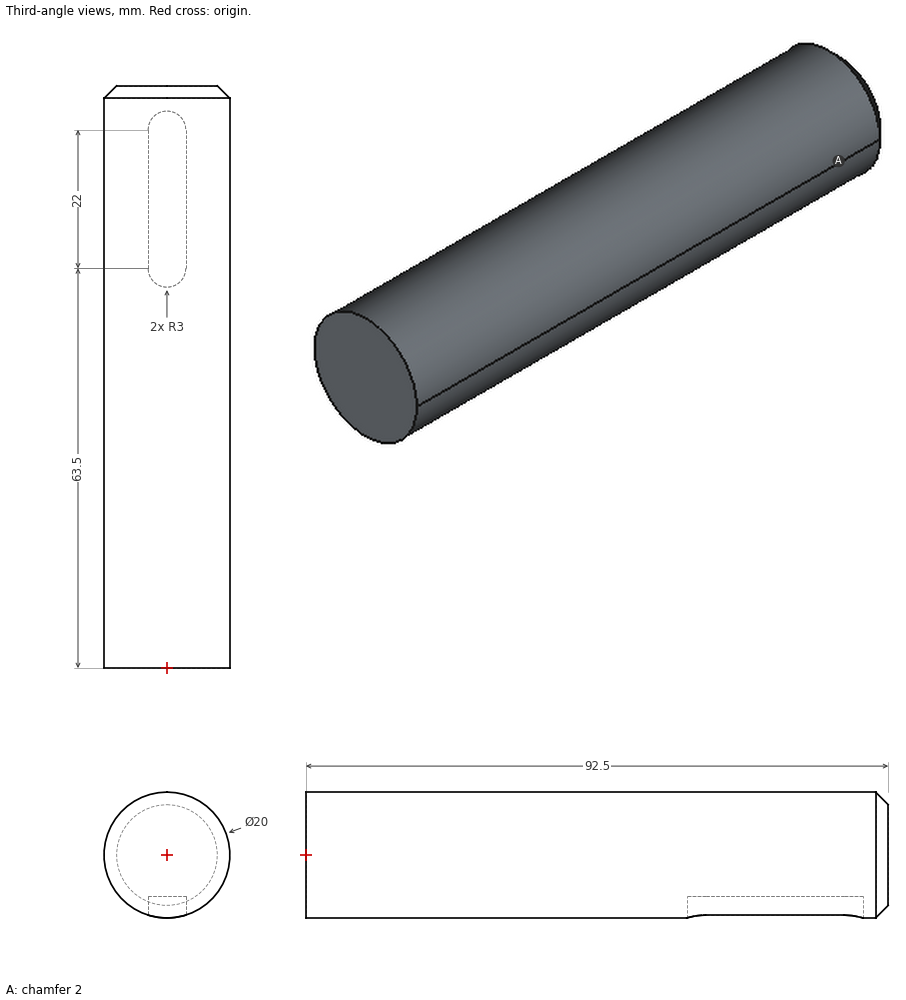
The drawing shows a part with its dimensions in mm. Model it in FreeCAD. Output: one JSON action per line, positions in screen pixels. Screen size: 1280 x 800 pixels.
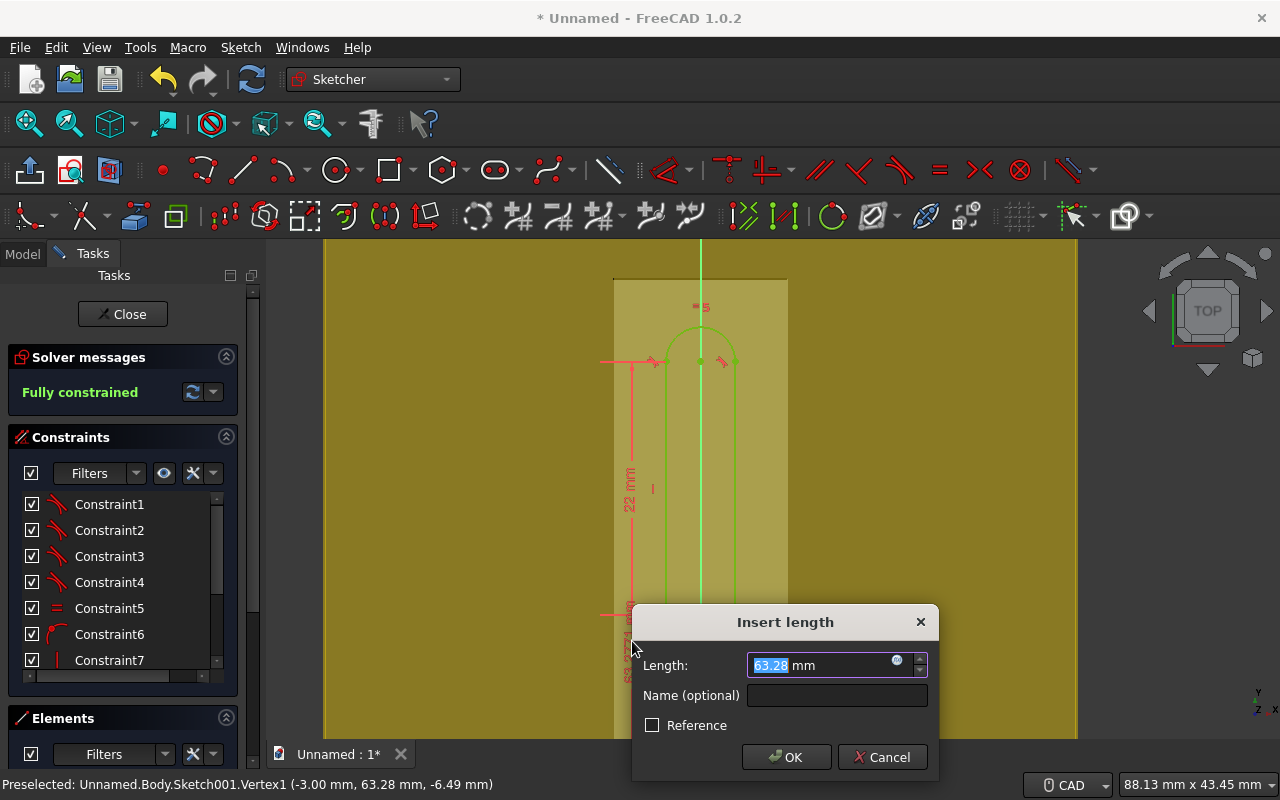
{"action": "type", "text": "63.5"}
{"action": "key", "text": "Return"}
{"action": "key", "text": "Escape"}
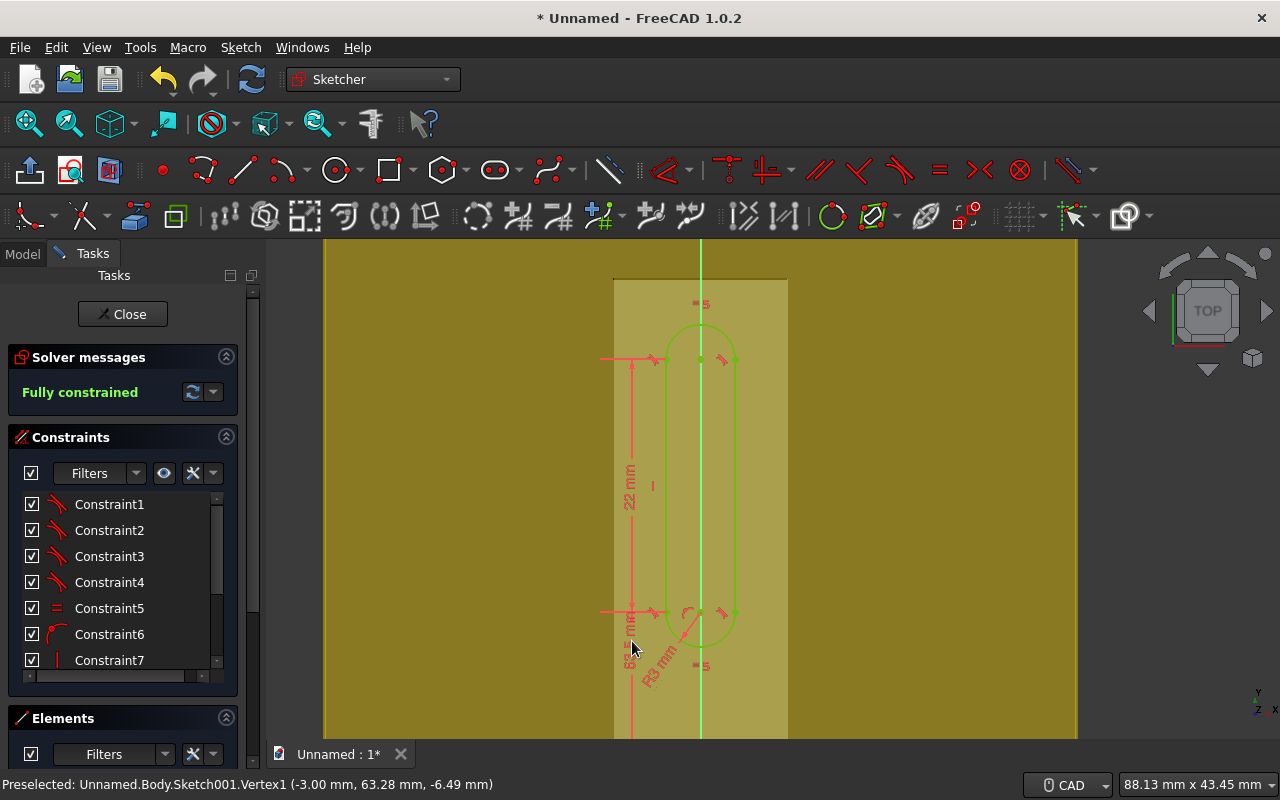
{"action": "left_click", "coordinate": [123, 314]}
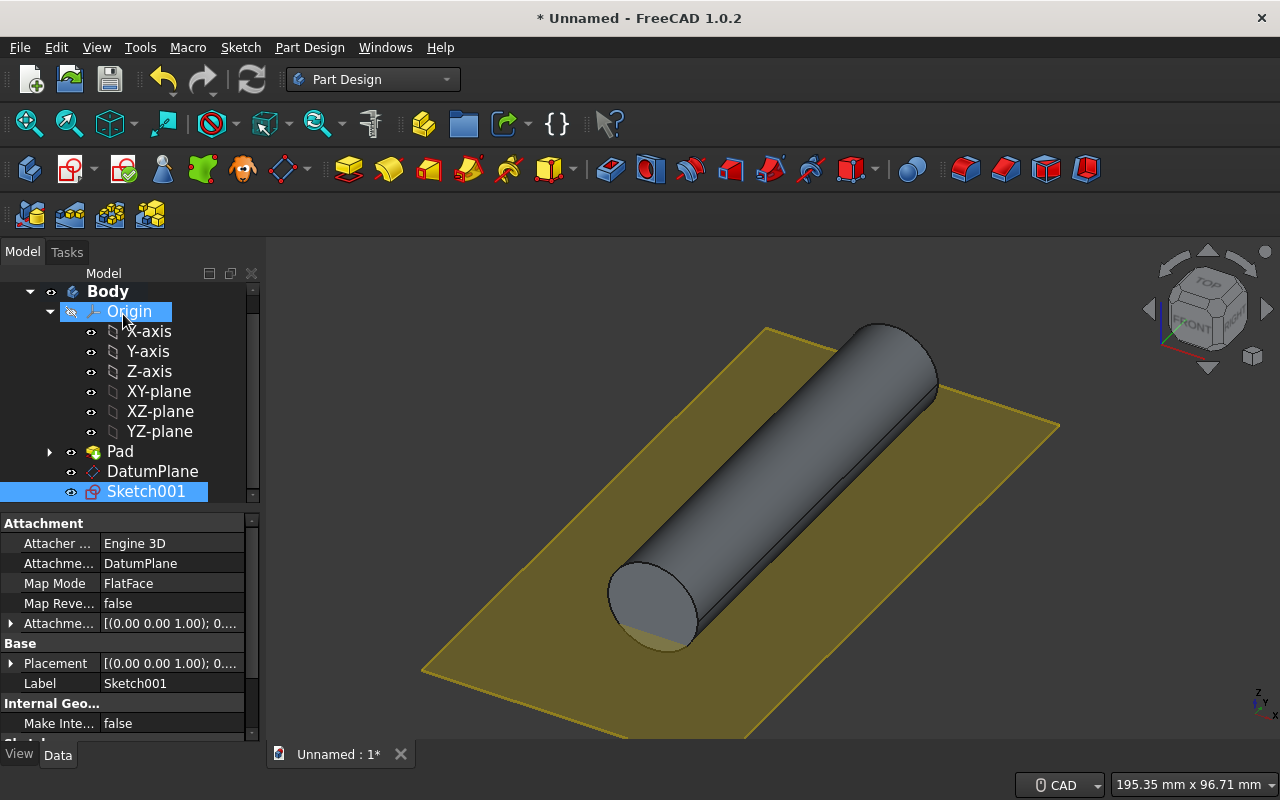
{"action": "left_click", "coordinate": [612, 170]}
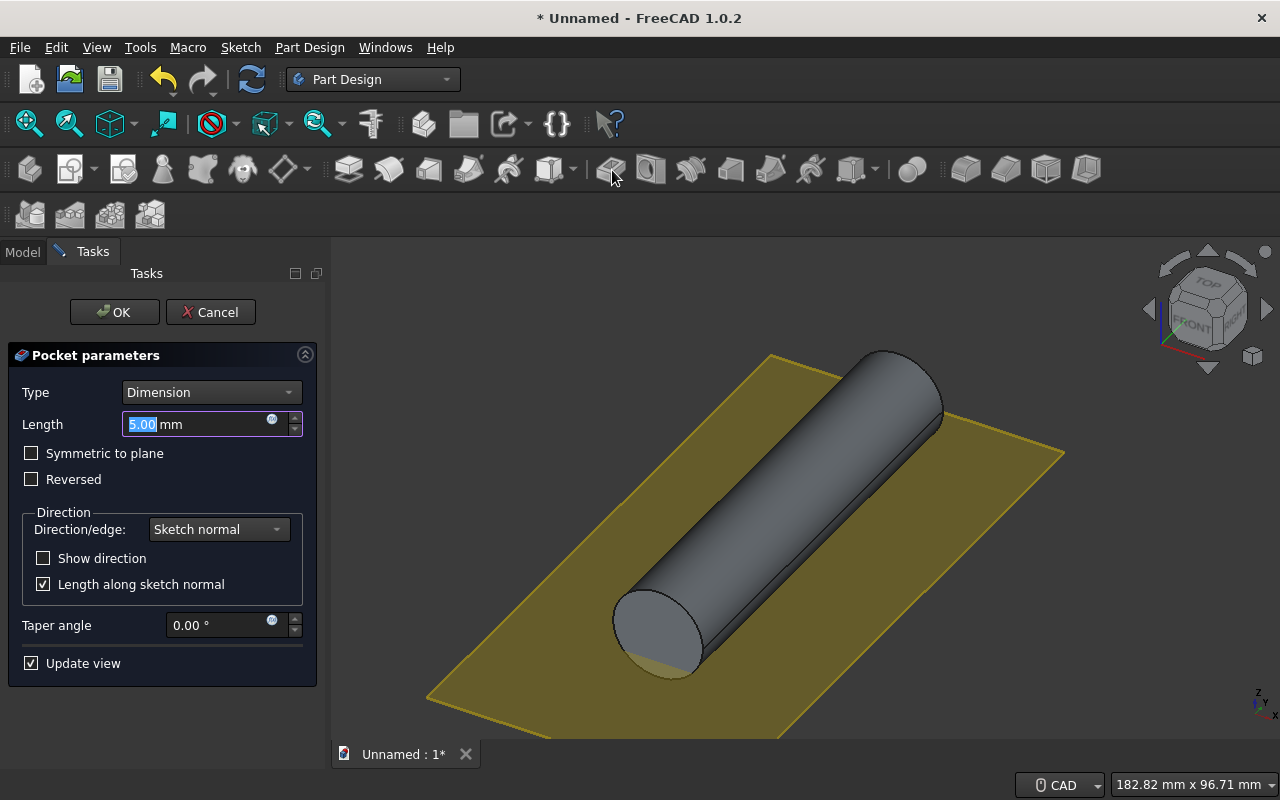
{"action": "left_click", "coordinate": [212, 392]}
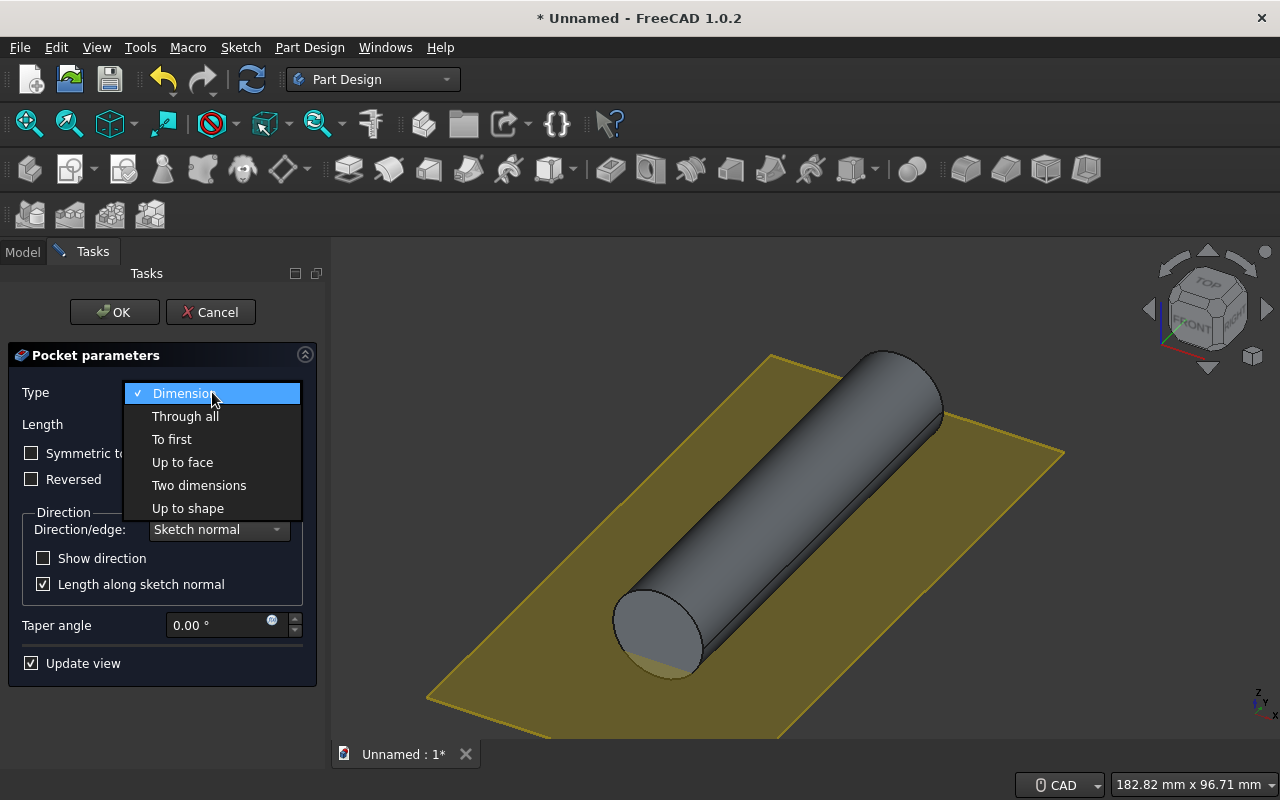
{"action": "left_click", "coordinate": [212, 416]}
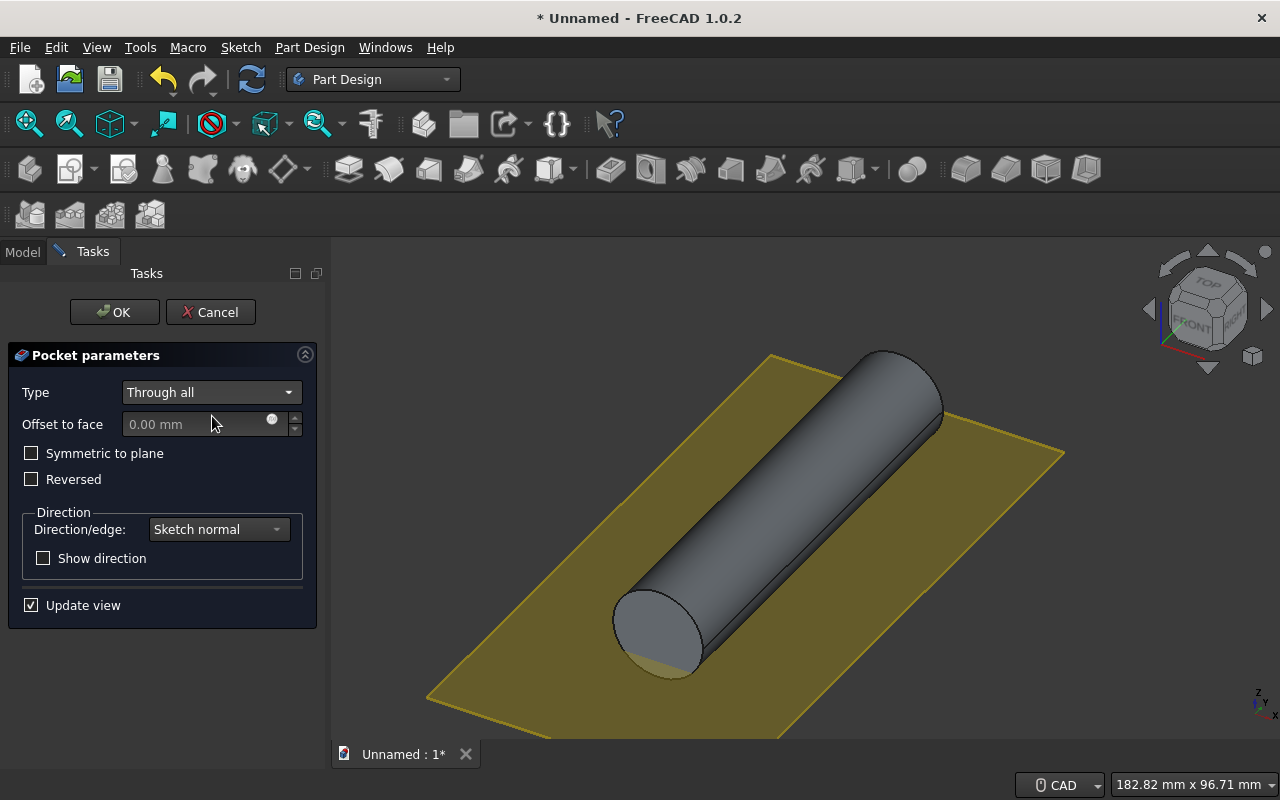
{"action": "left_click", "coordinate": [115, 312]}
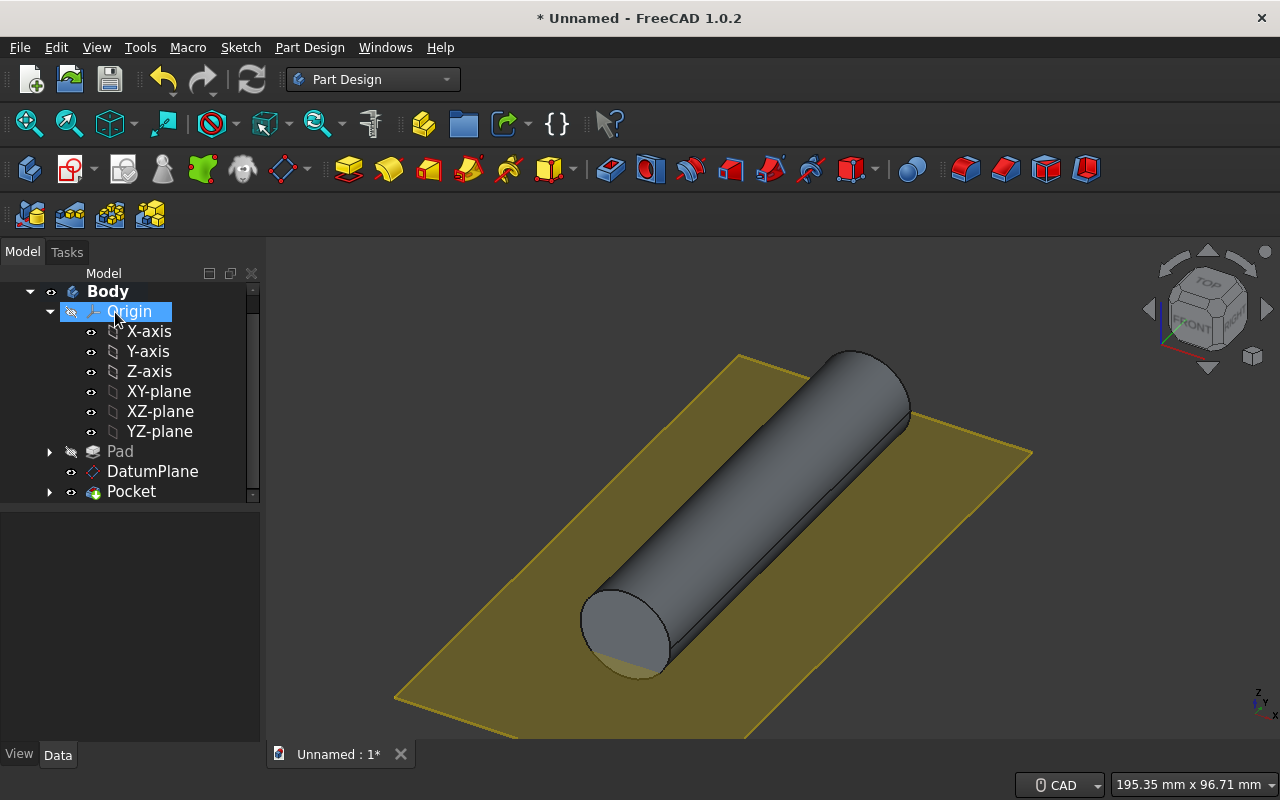
{"action": "left_click", "coordinate": [116, 472]}
{"action": "key", "text": "space"}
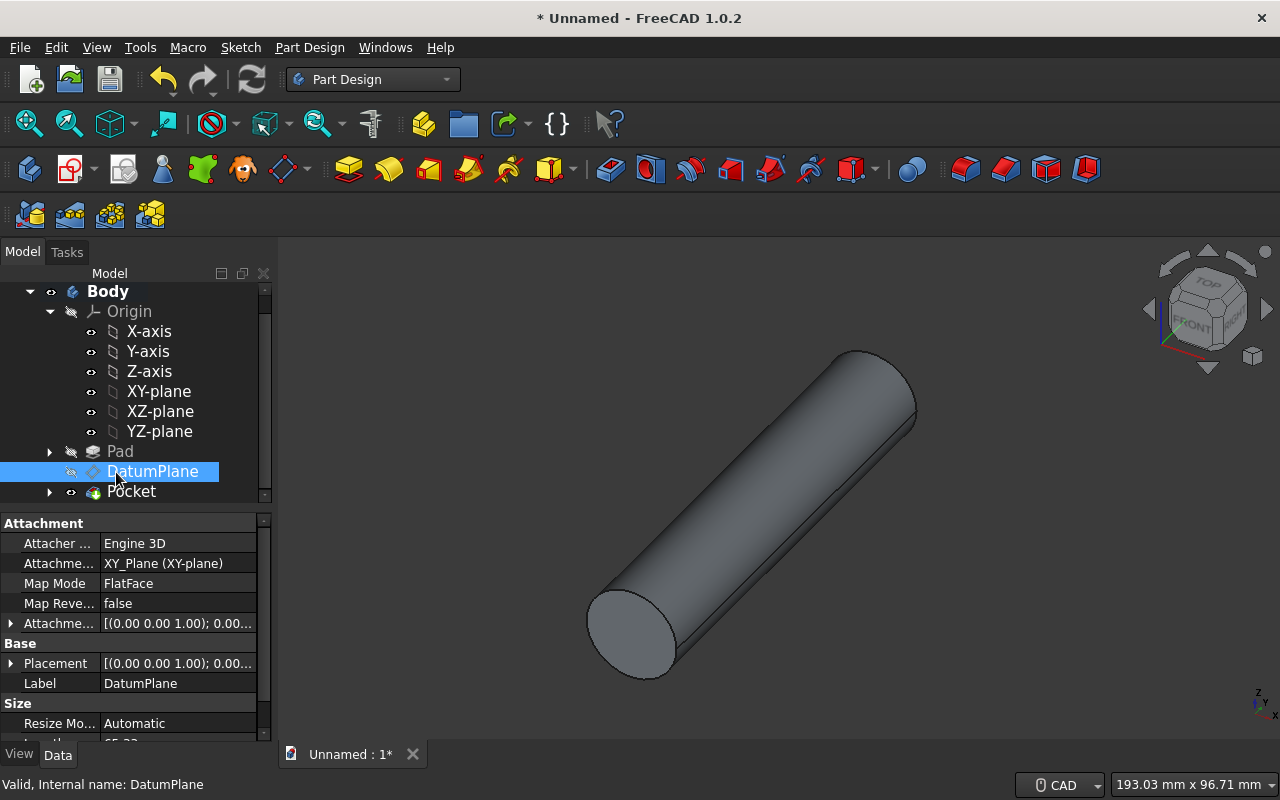
{"action": "key", "text": "0"}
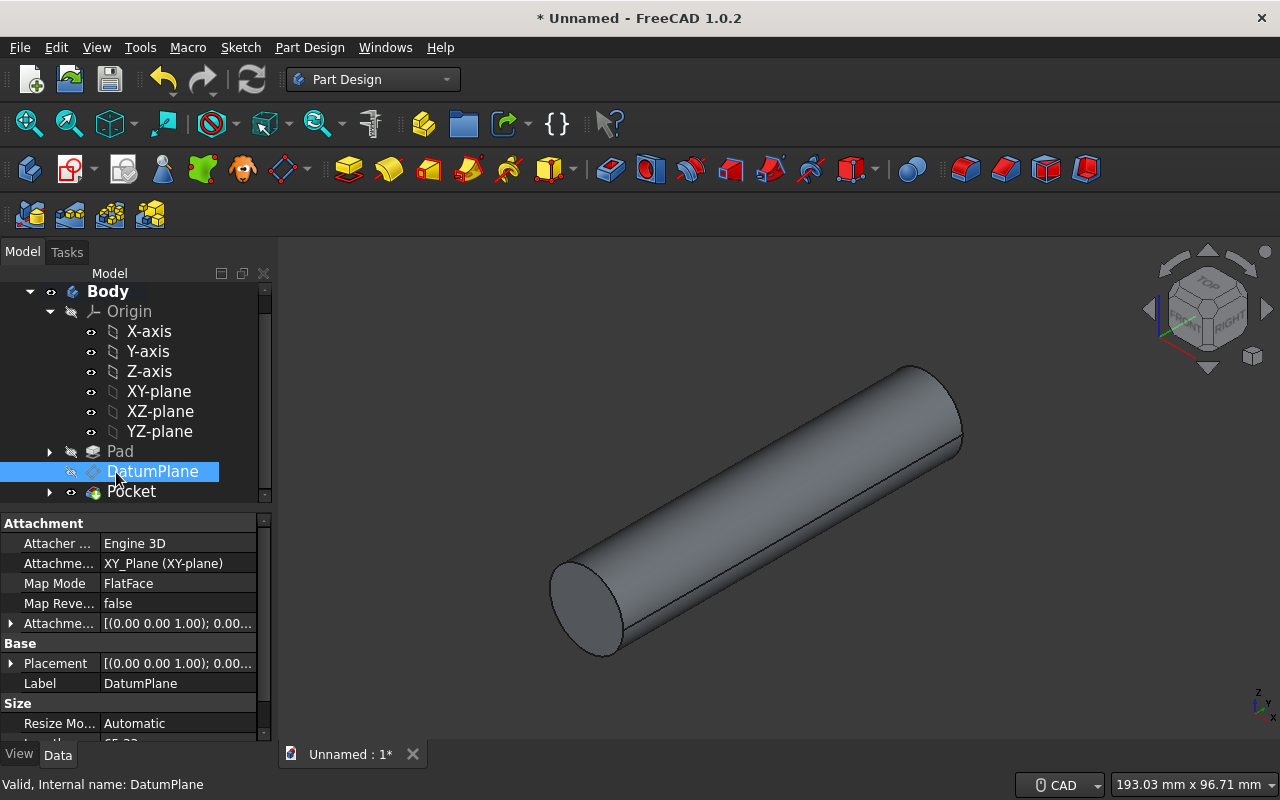
{"action": "key", "text": "2"}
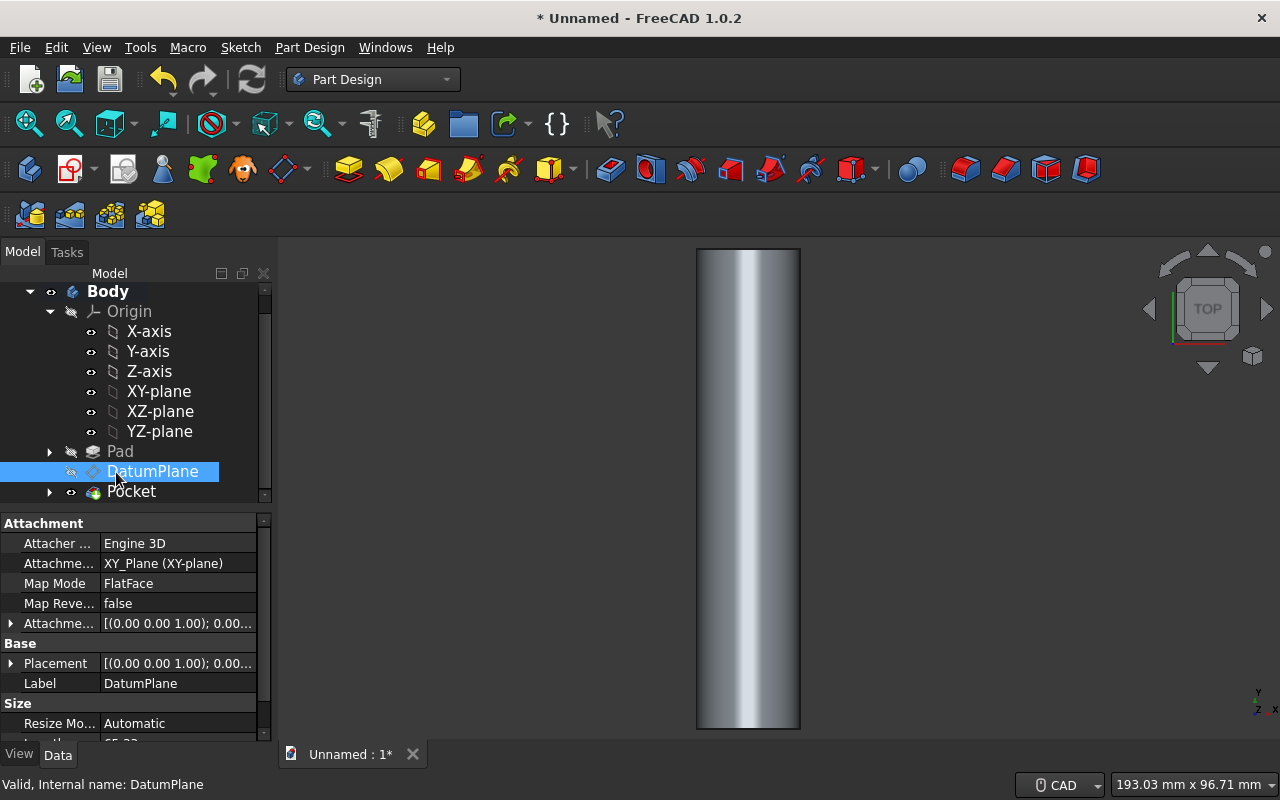
{"action": "key", "text": "1"}